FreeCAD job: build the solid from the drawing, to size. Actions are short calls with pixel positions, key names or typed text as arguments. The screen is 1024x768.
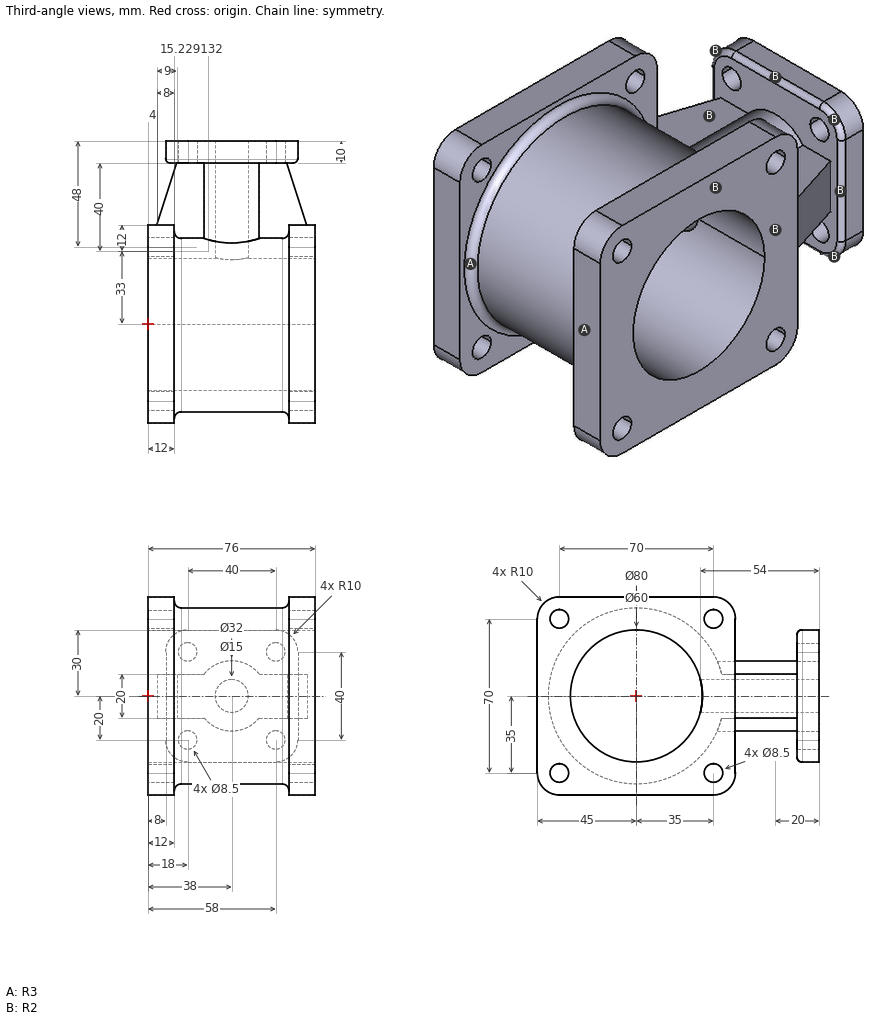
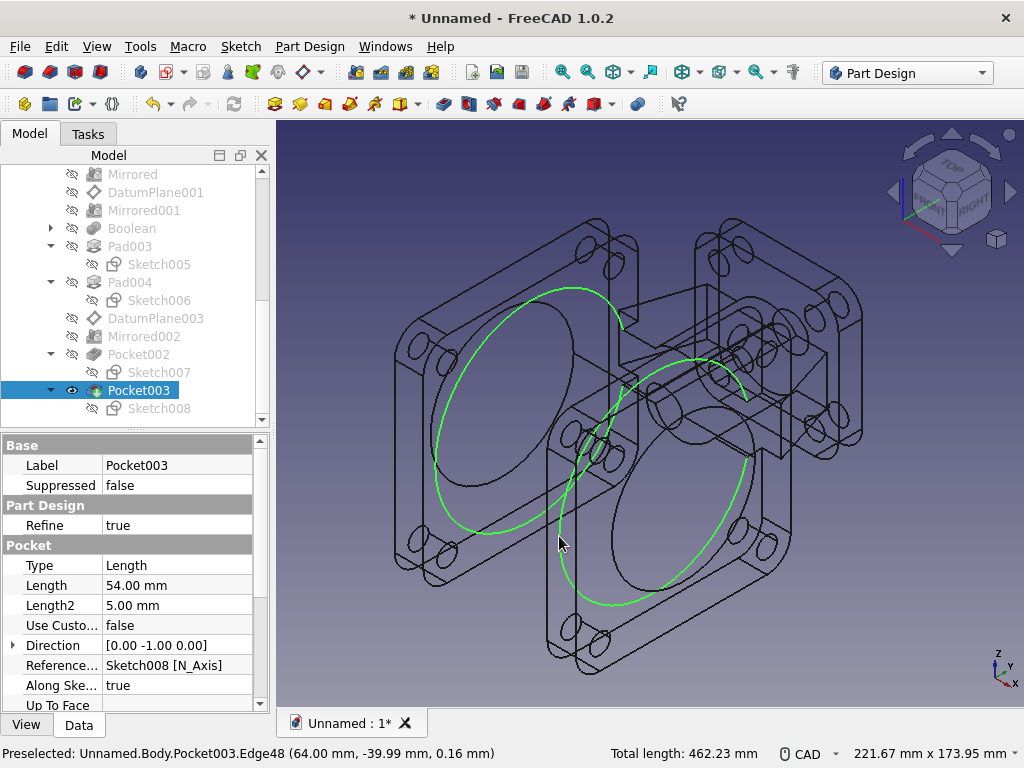
key(v)
key(1)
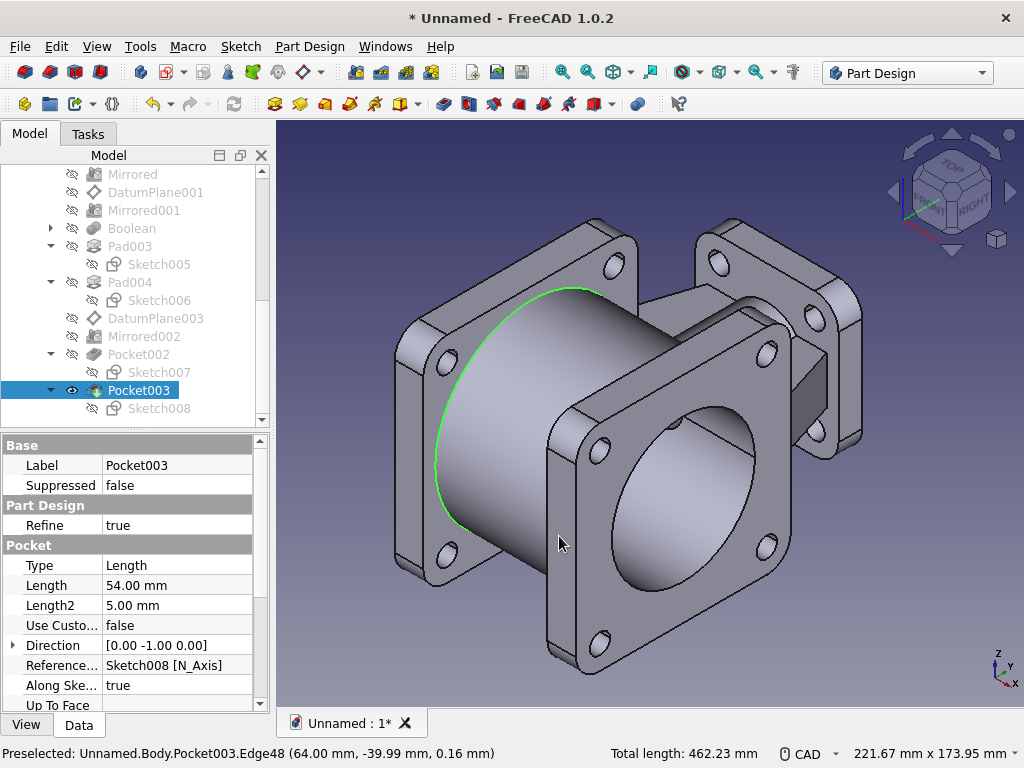
click(25, 72)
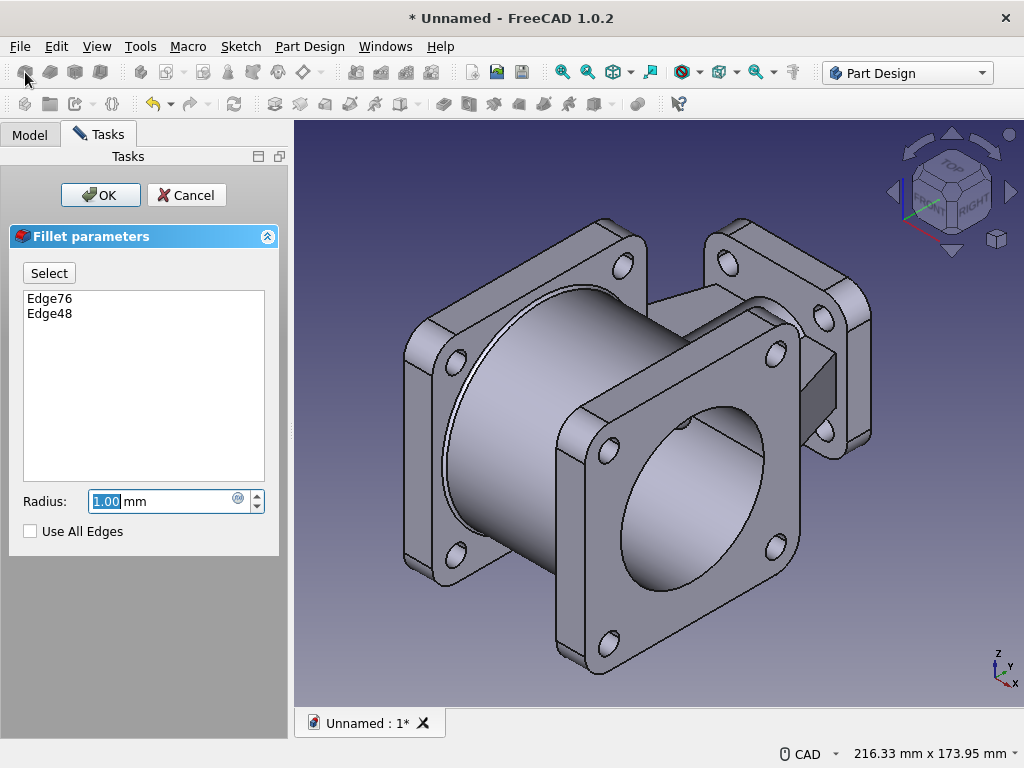
text(3)
key(Tab)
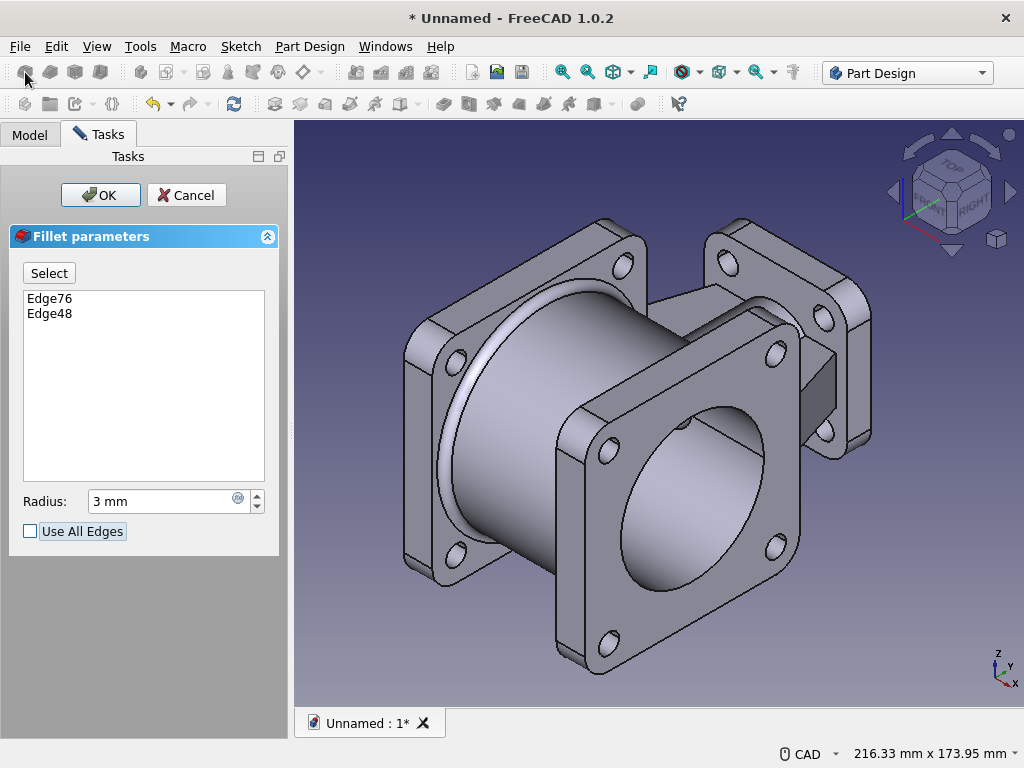
click(101, 195)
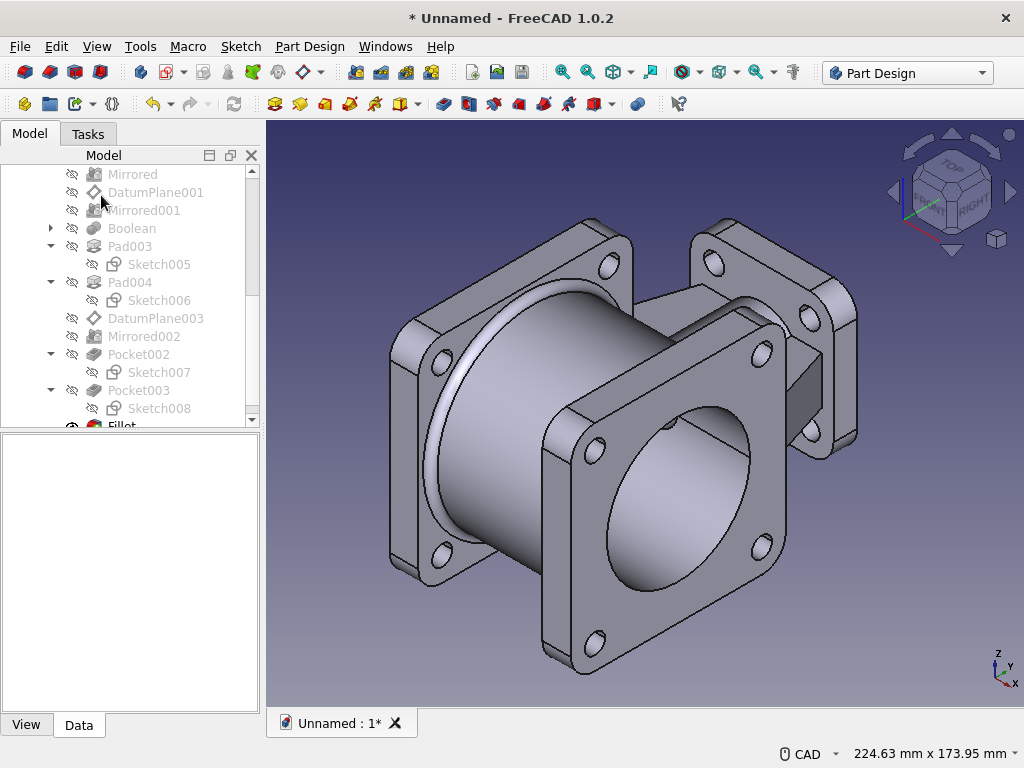
click(697, 233)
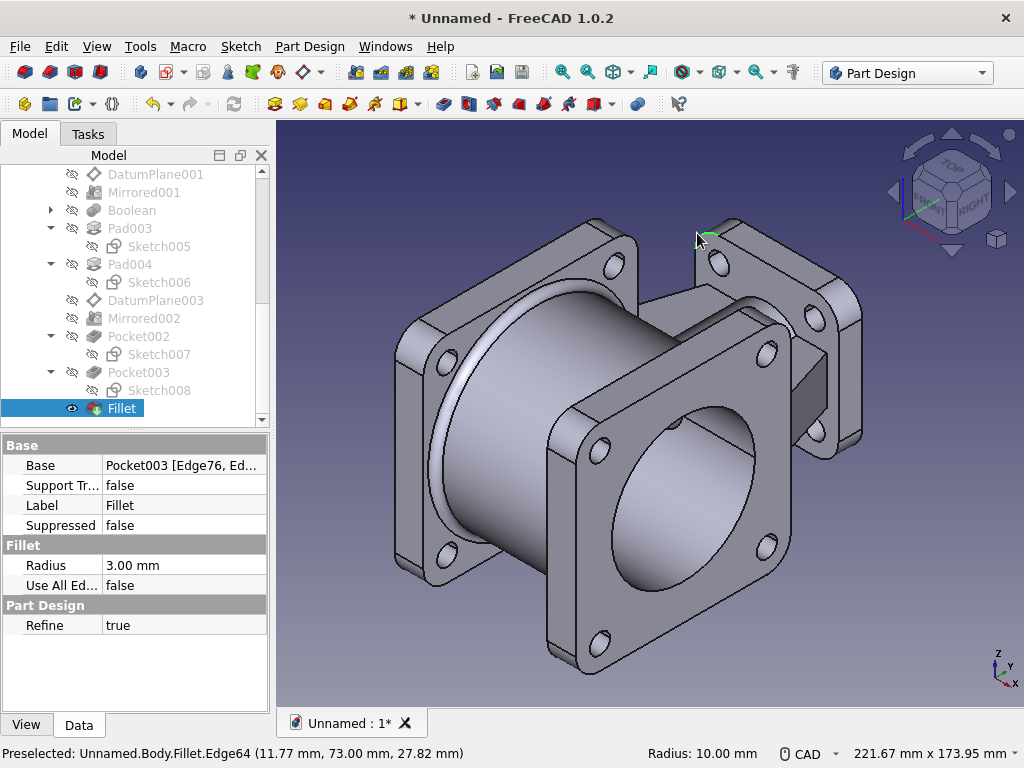
click(832, 457, ctrl)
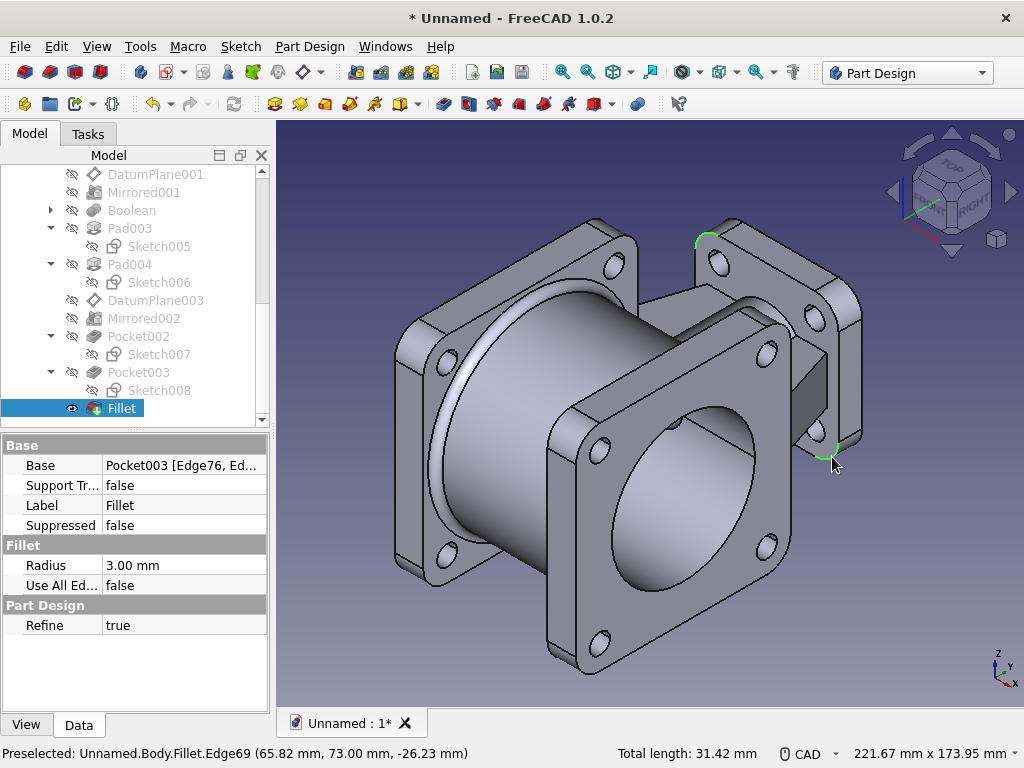
click(839, 386, ctrl)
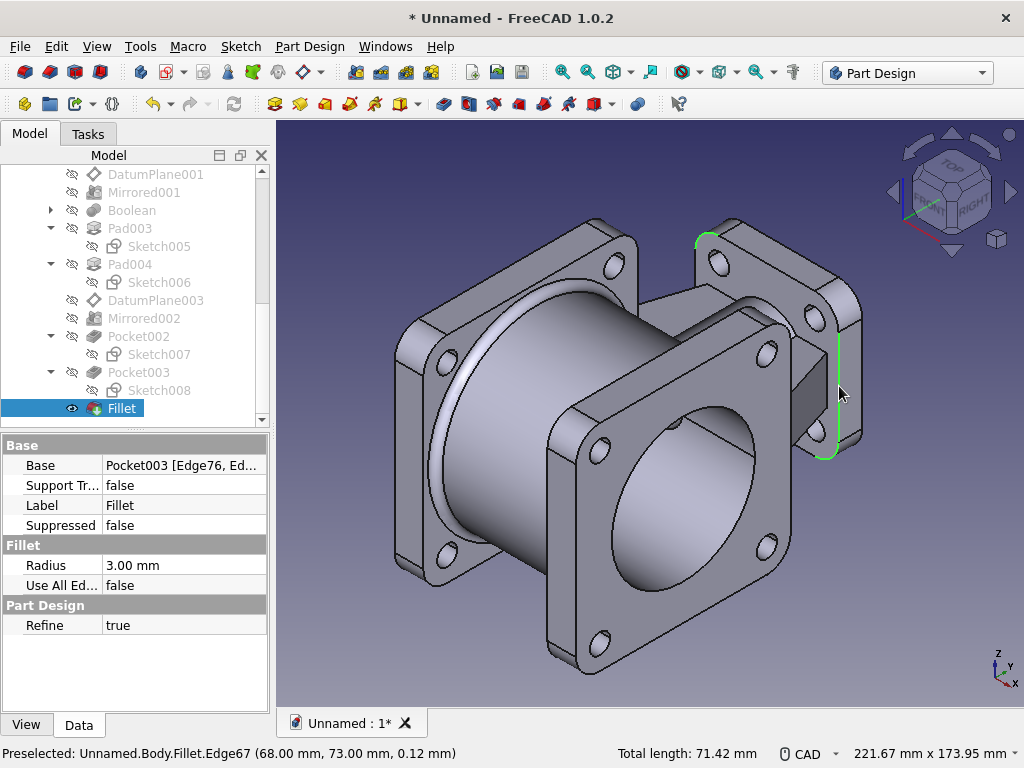
click(832, 308, ctrl)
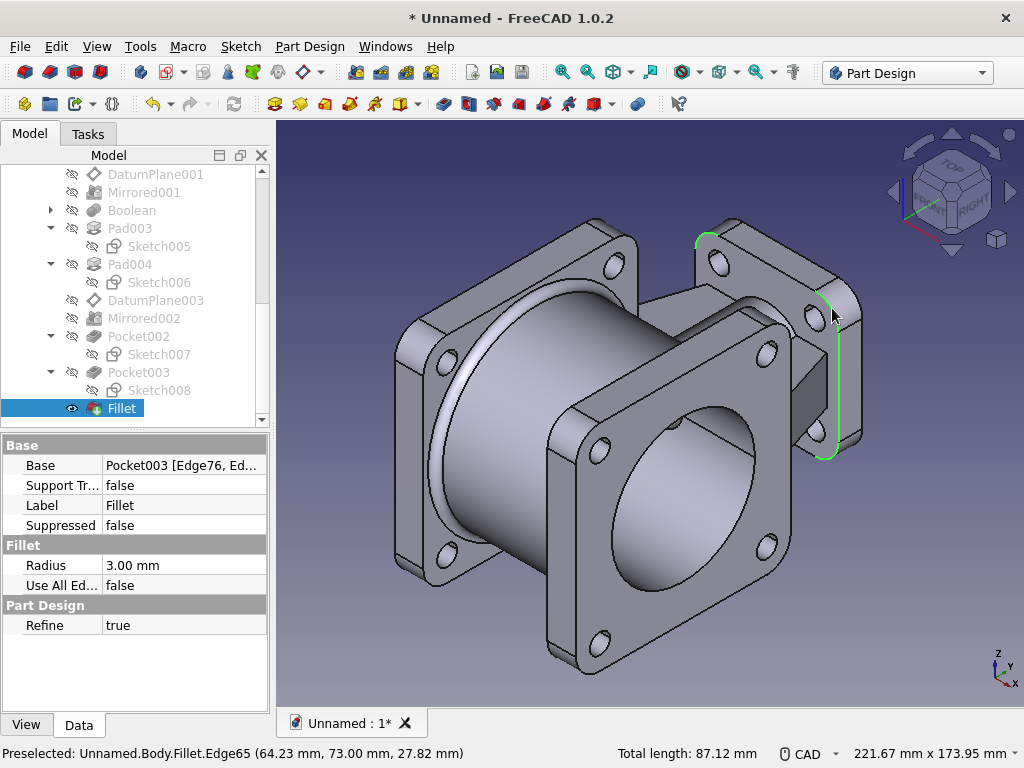
click(767, 262, ctrl)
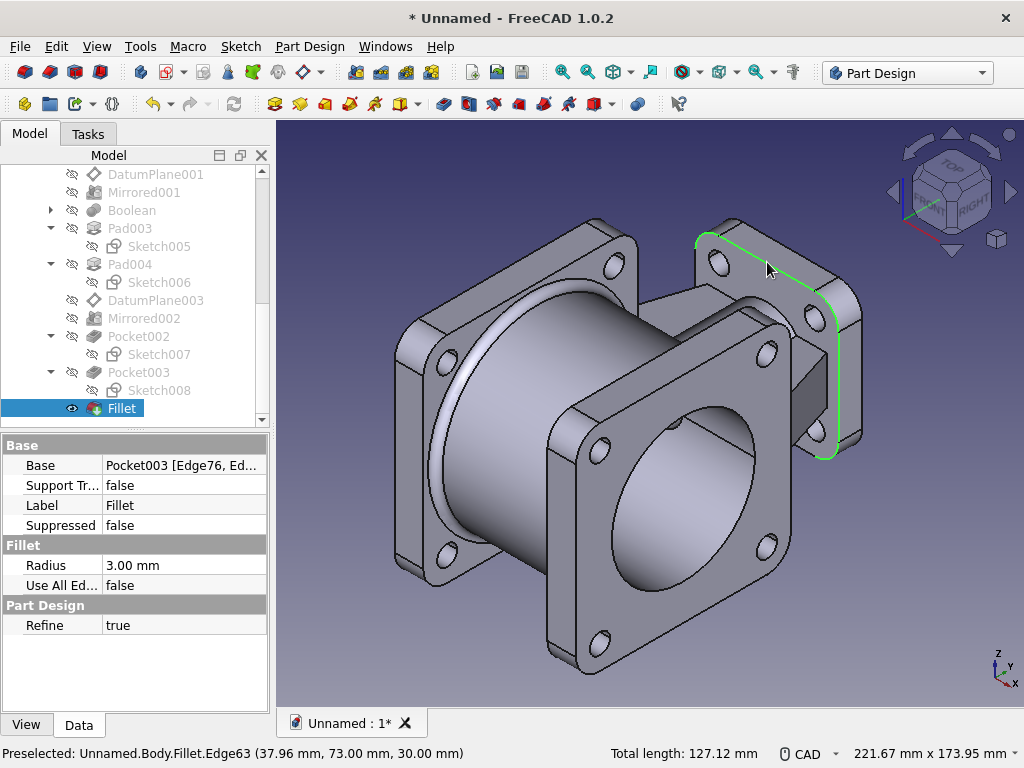
key(2)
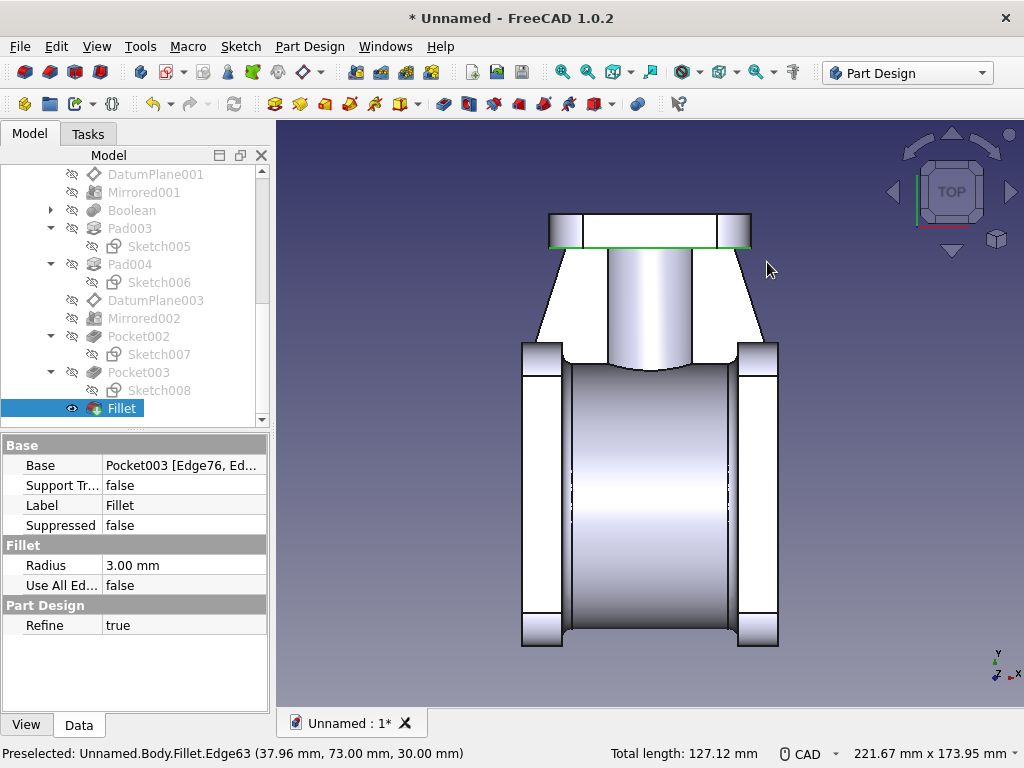
key(0)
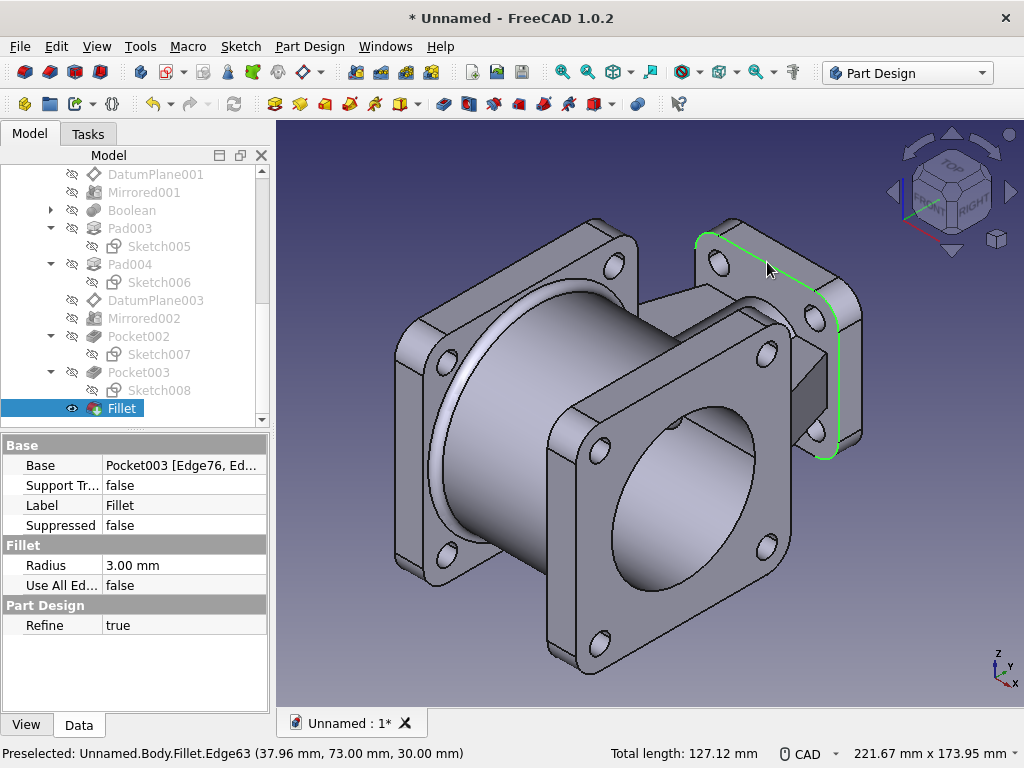
key(1)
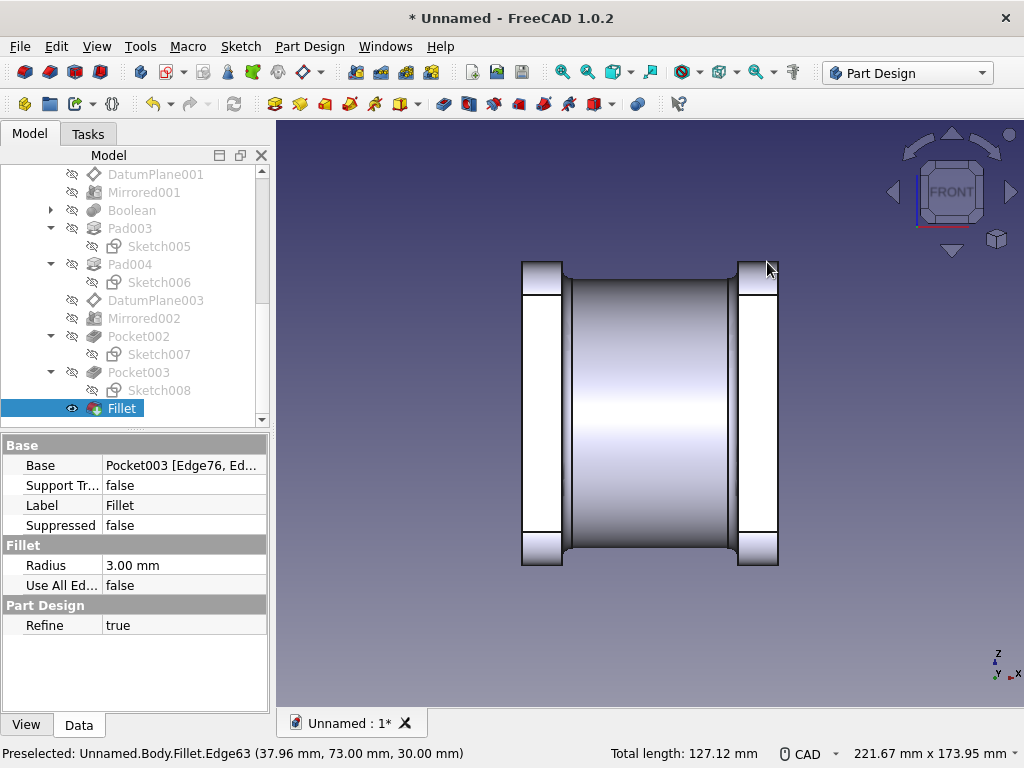
key(3)